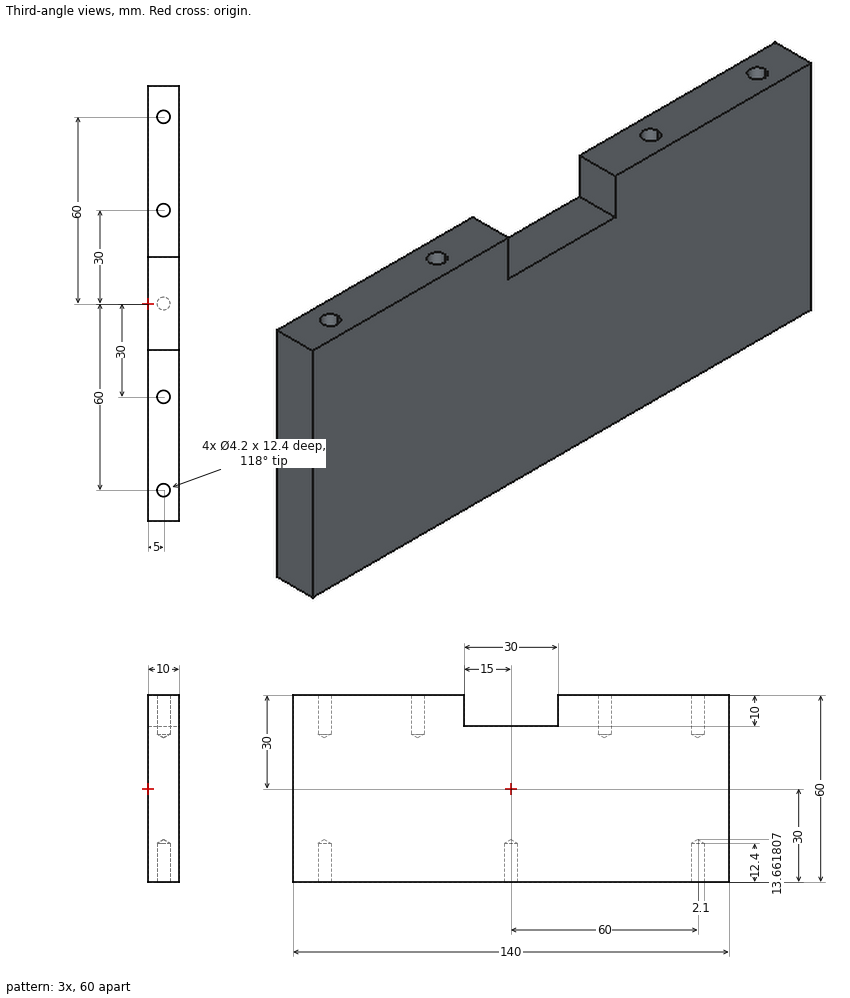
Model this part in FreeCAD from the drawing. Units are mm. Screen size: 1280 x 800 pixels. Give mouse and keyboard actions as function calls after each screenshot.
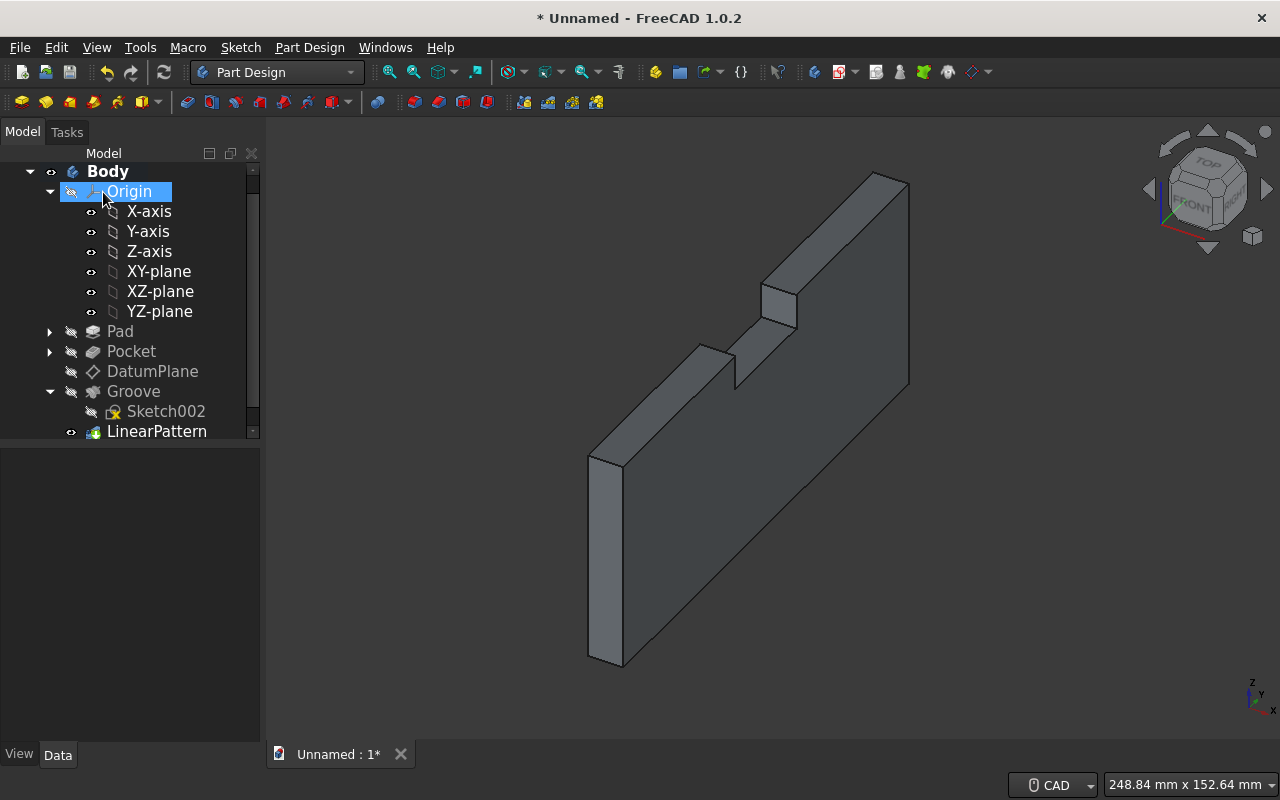
click(694, 373)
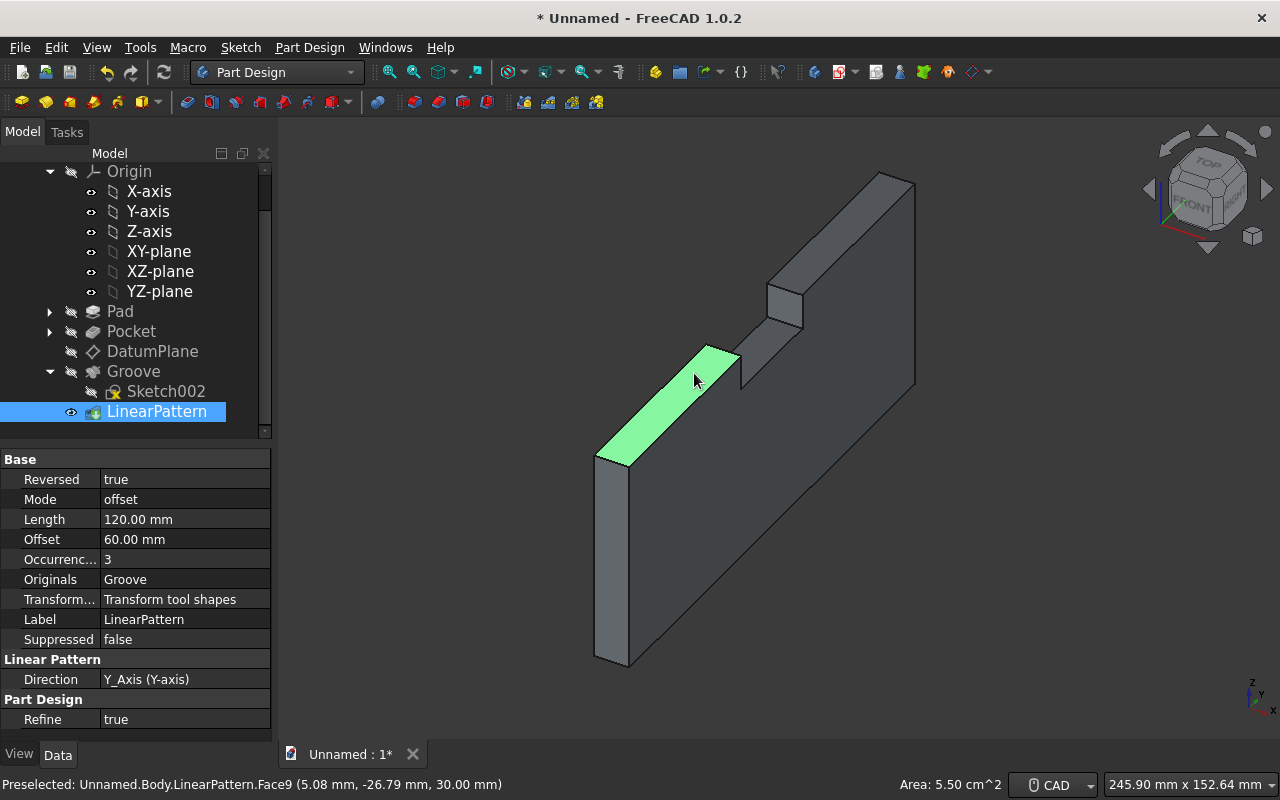
click(840, 72)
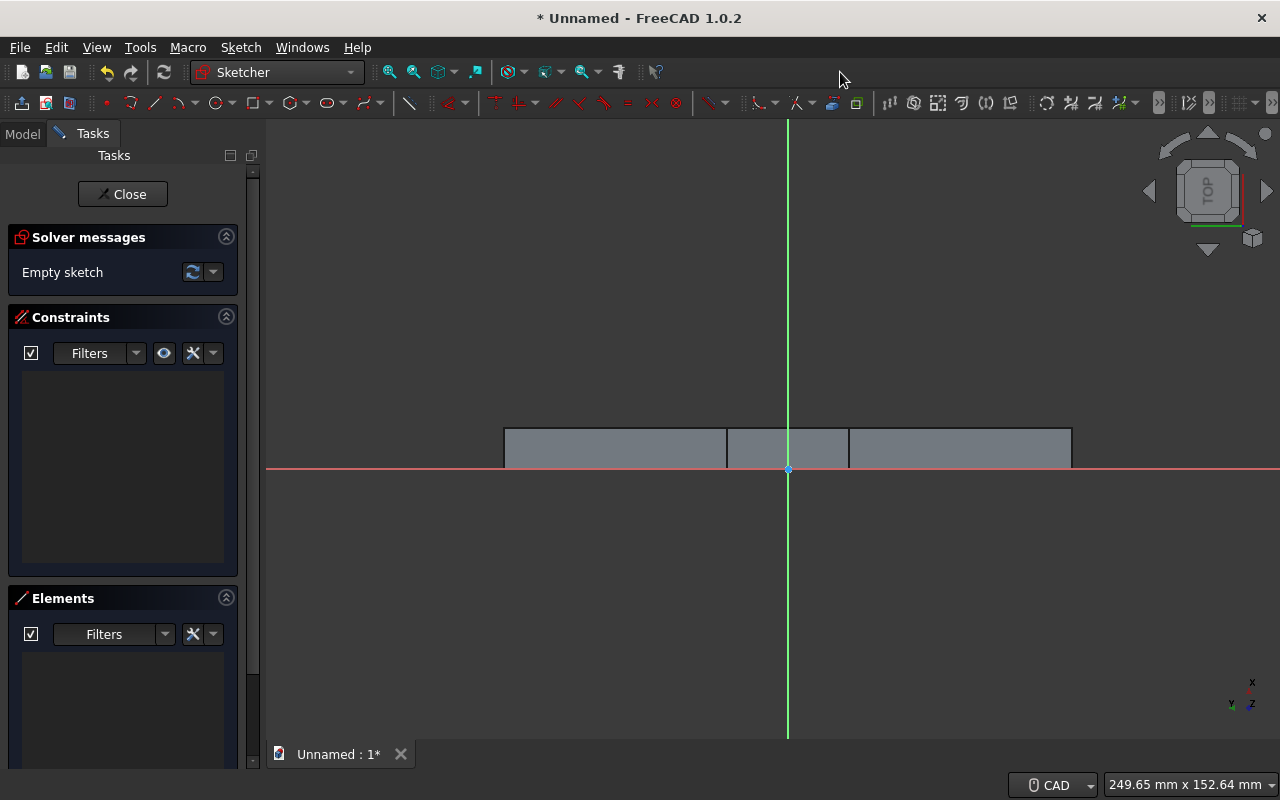
key(g)
key(c)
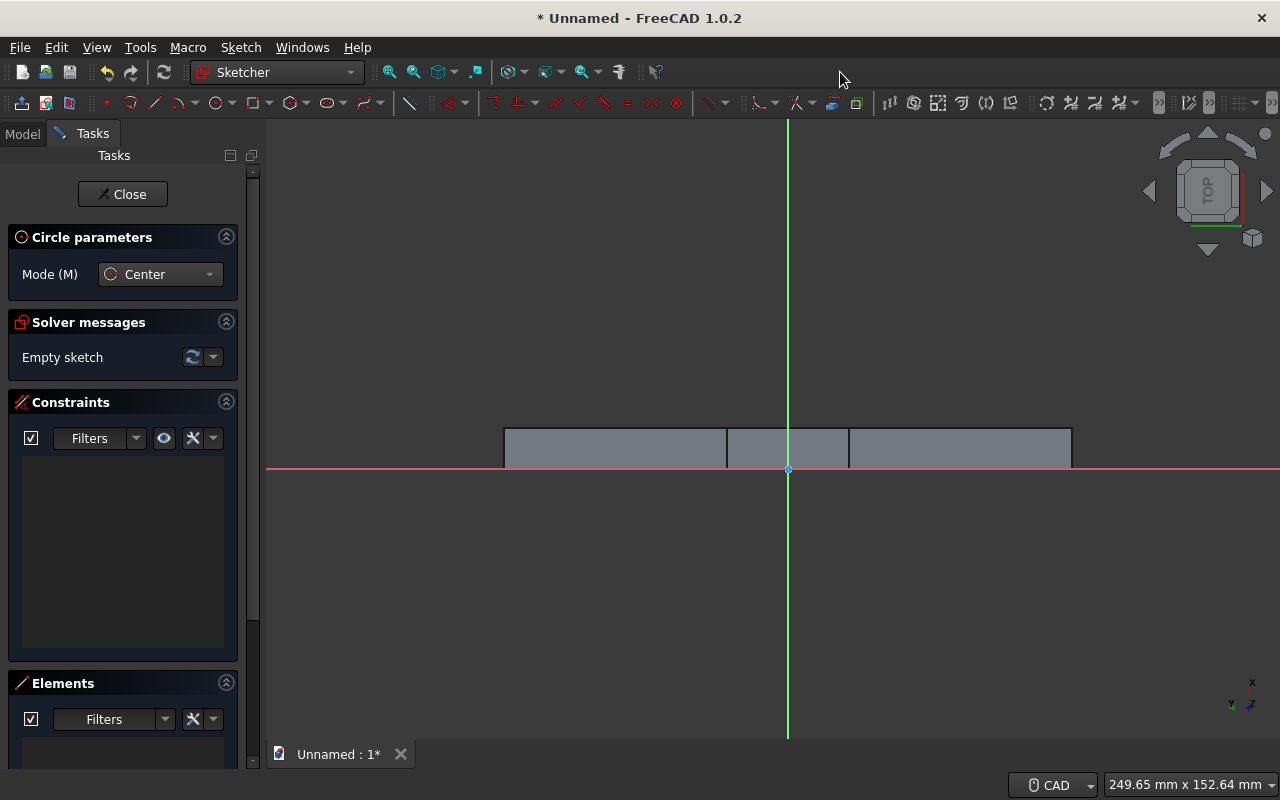
scroll(1032, 449, up, 5)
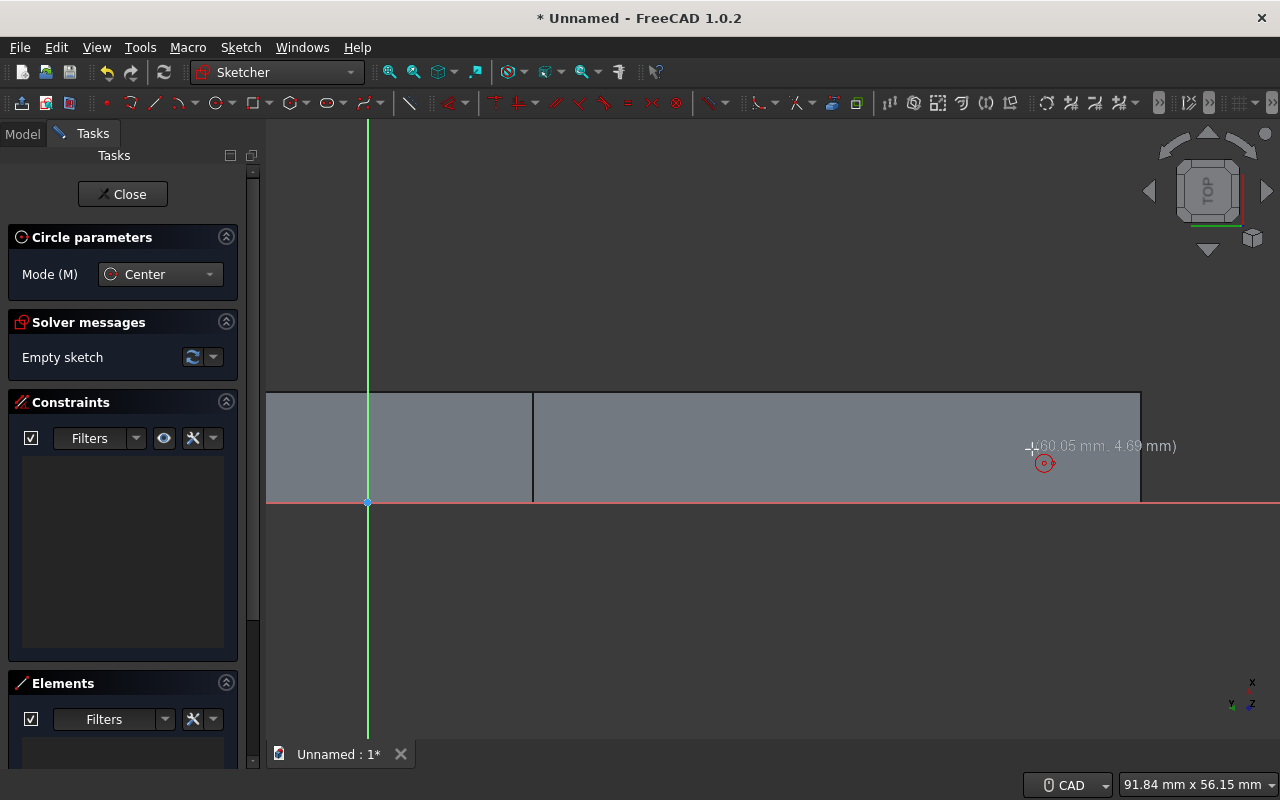
click(1030, 447)
move(1047, 431)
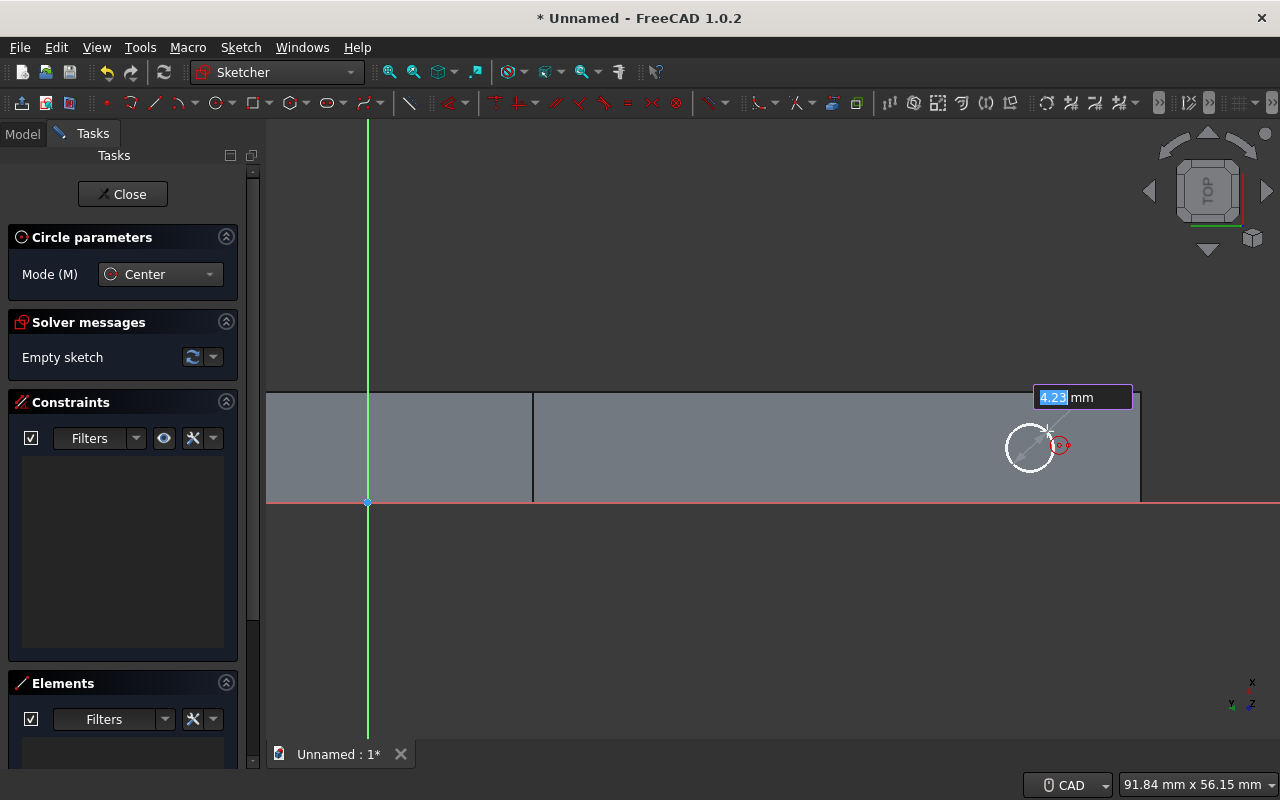
text(4.2)
key(Return)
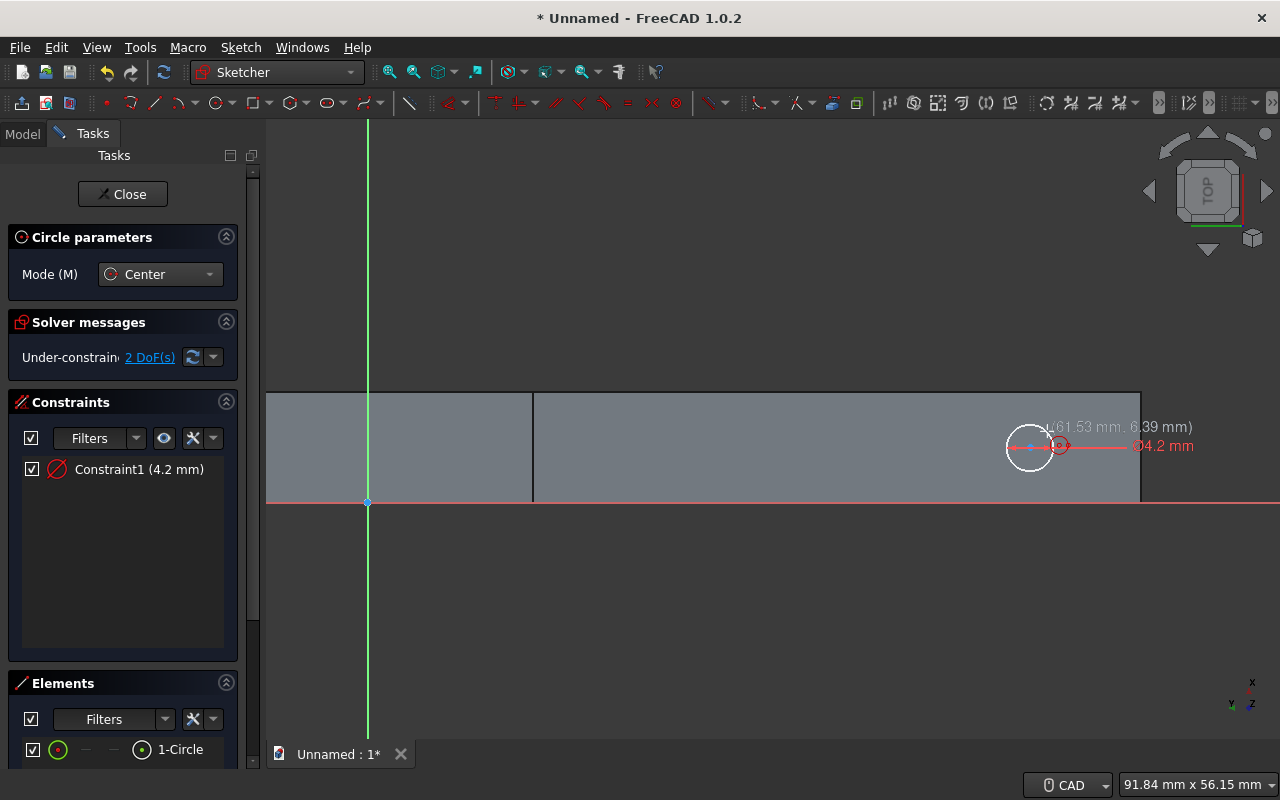
click(699, 447)
move(715, 431)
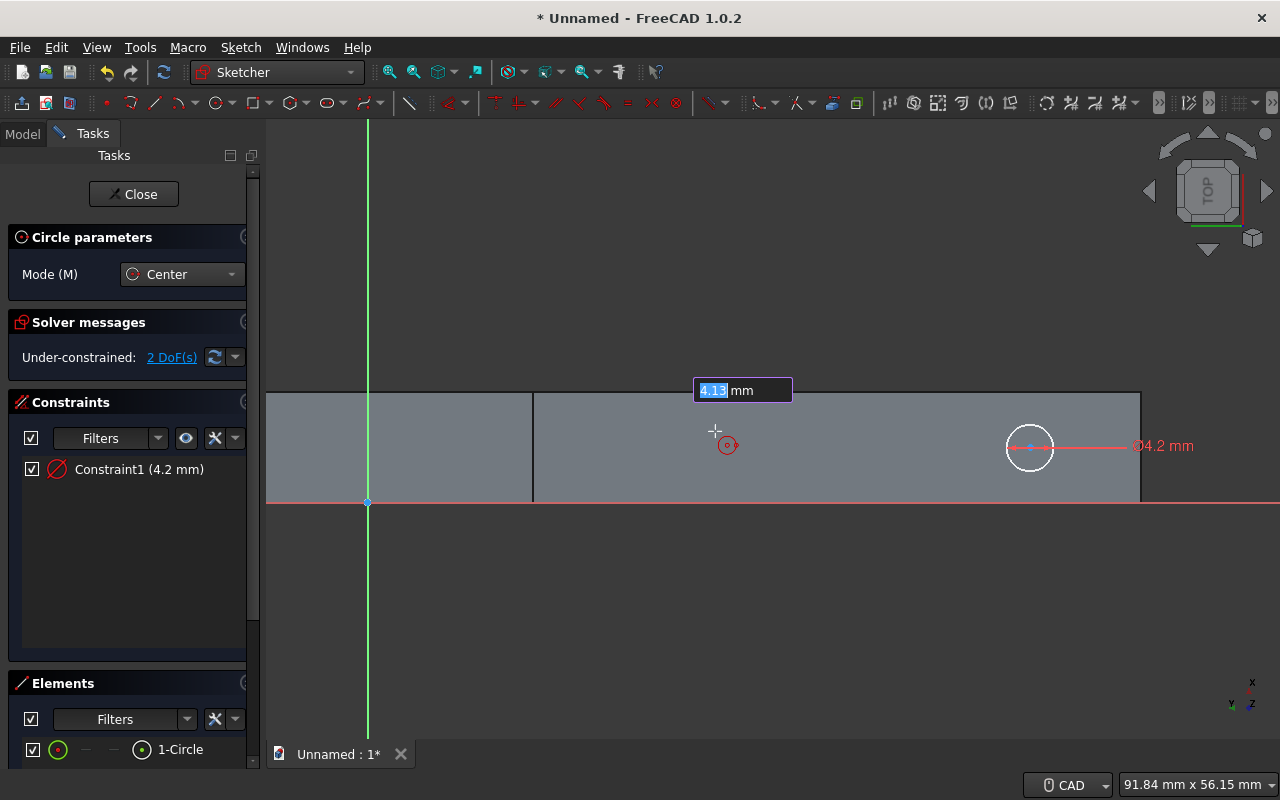
text(4.2)
key(Return)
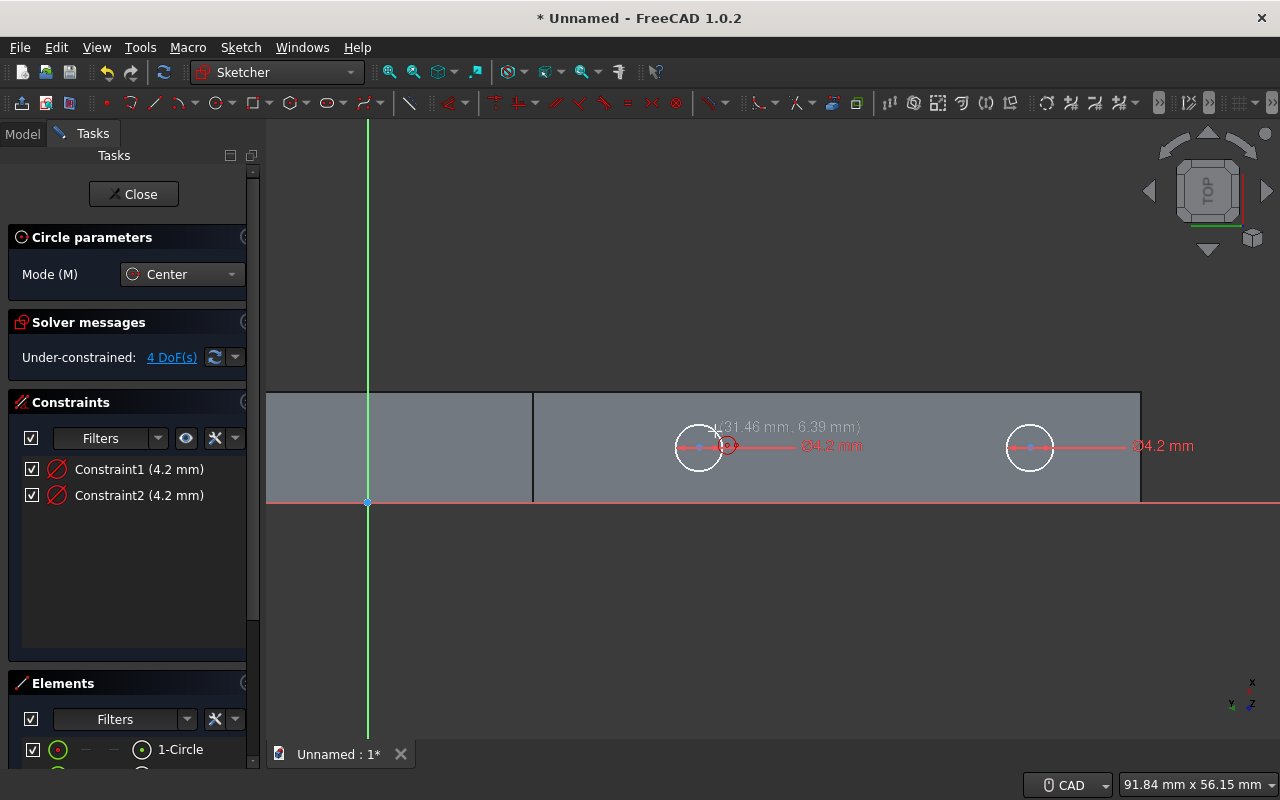
scroll(979, 401, down, 4)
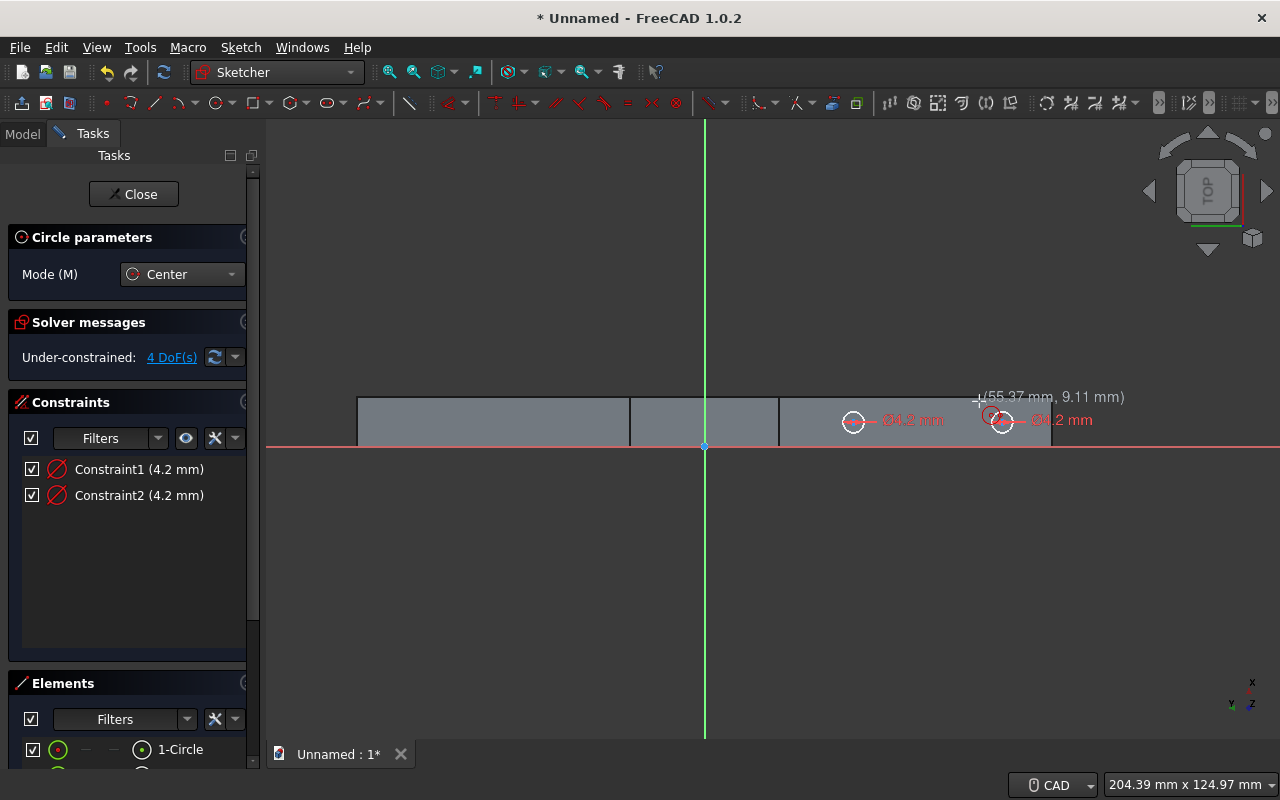
scroll(556, 422, up, 4)